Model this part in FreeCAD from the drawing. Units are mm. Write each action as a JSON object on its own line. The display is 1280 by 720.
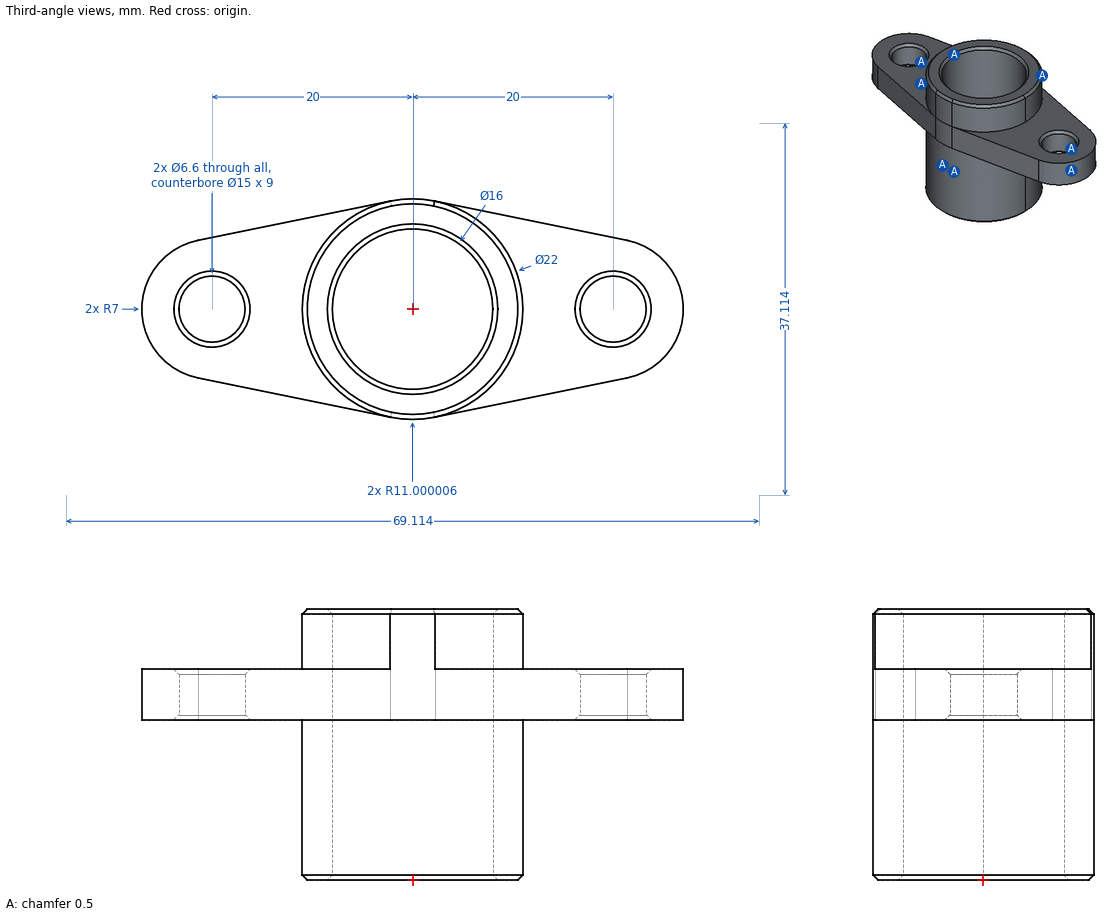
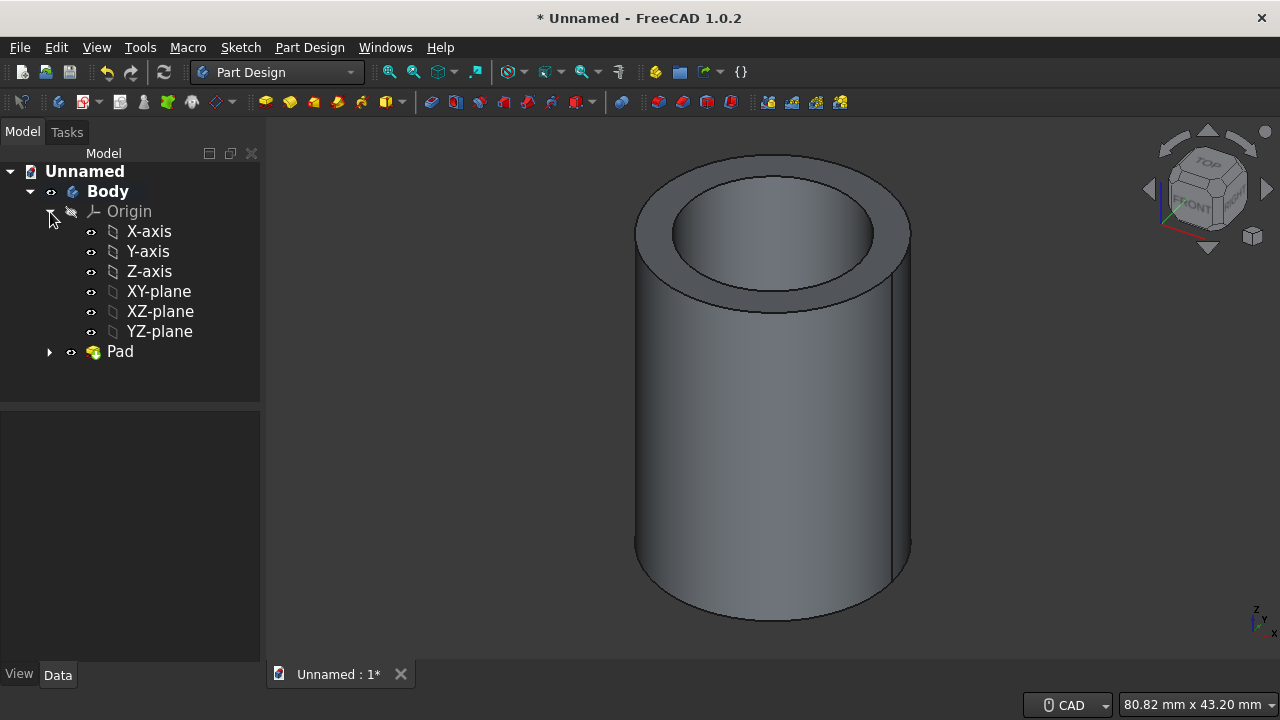
{"action": "left_click", "coordinate": [136, 292]}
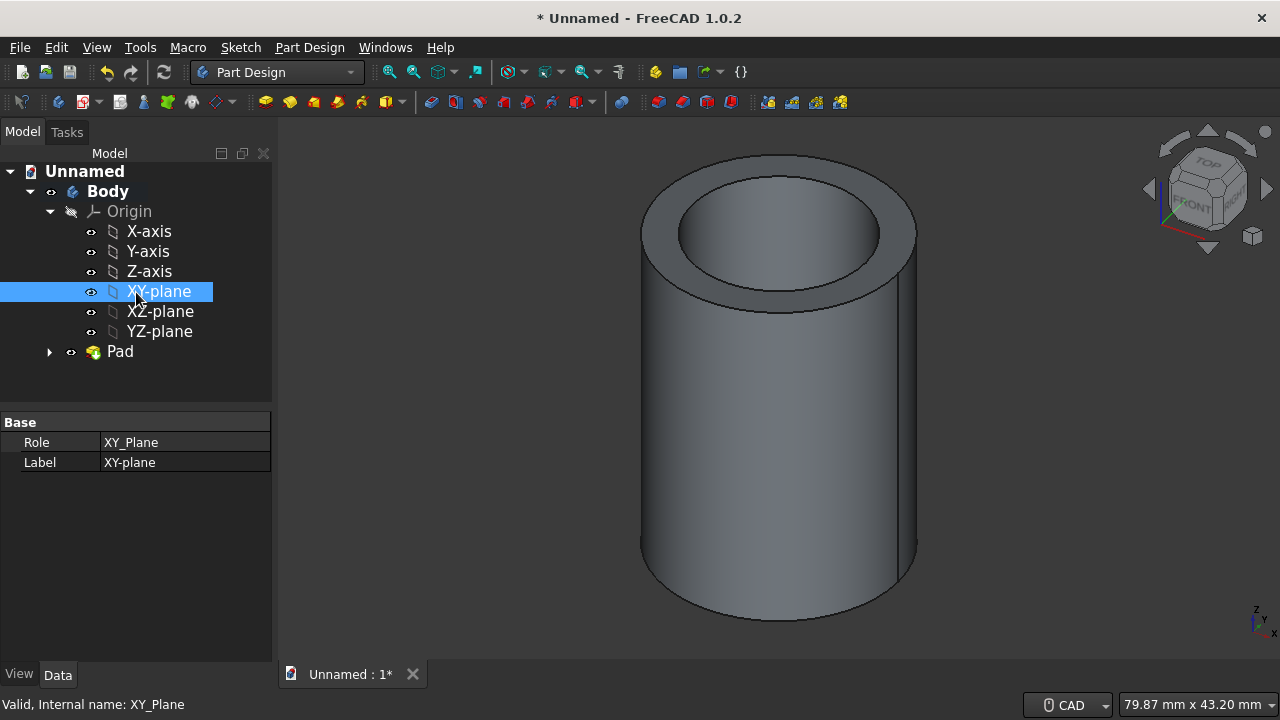
{"action": "left_click", "coordinate": [216, 102]}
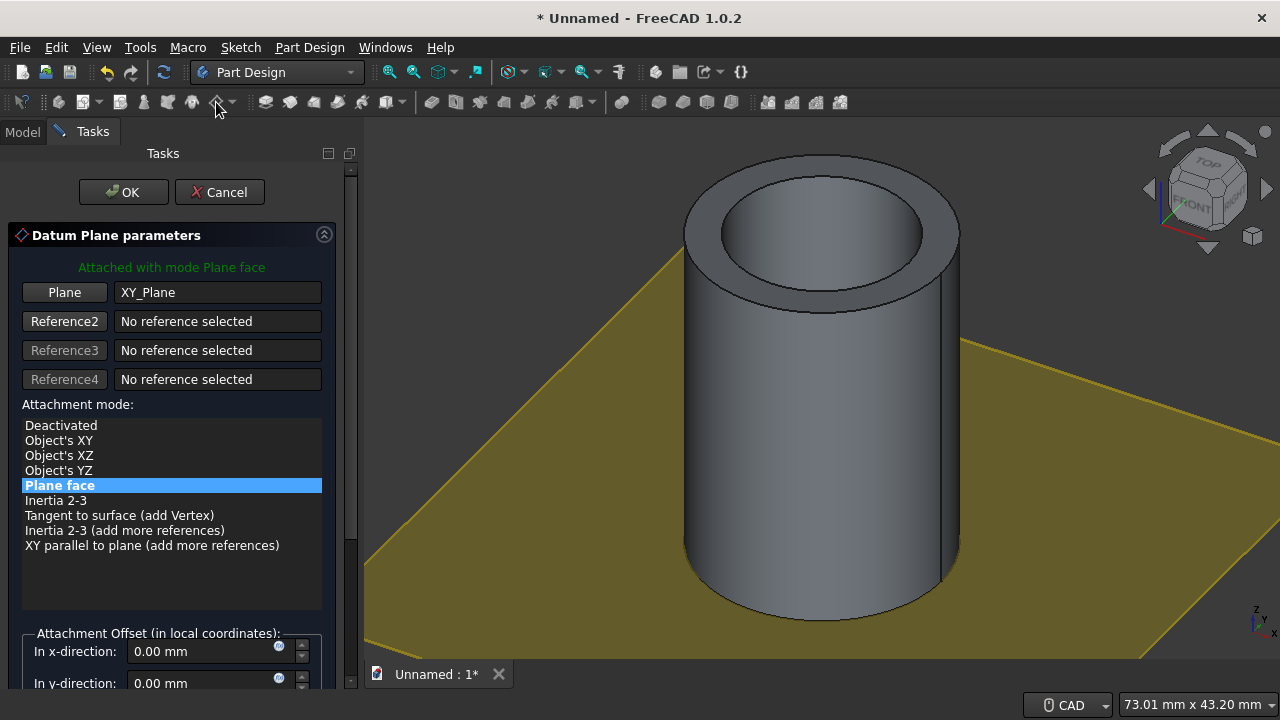
{"action": "scroll", "coordinate": [351, 426], "scroll_direction": "down", "scroll_amount": 2}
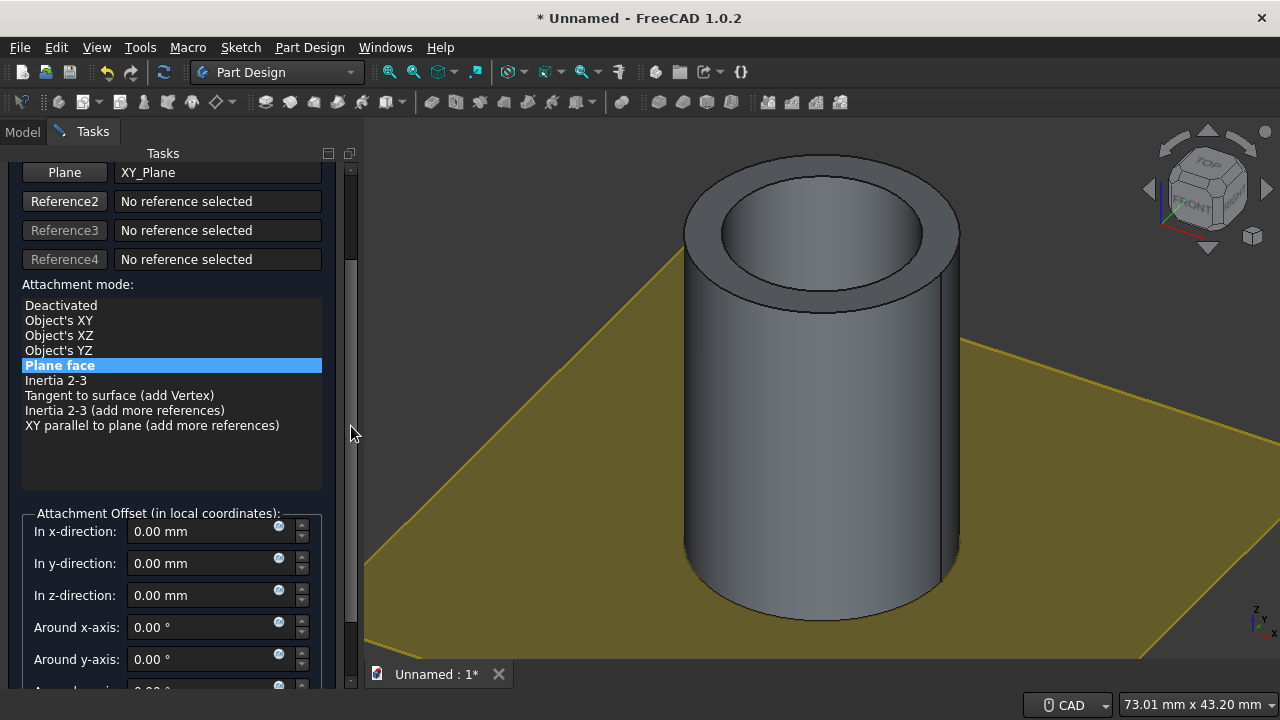
{"action": "triple_click", "coordinate": [210, 595]}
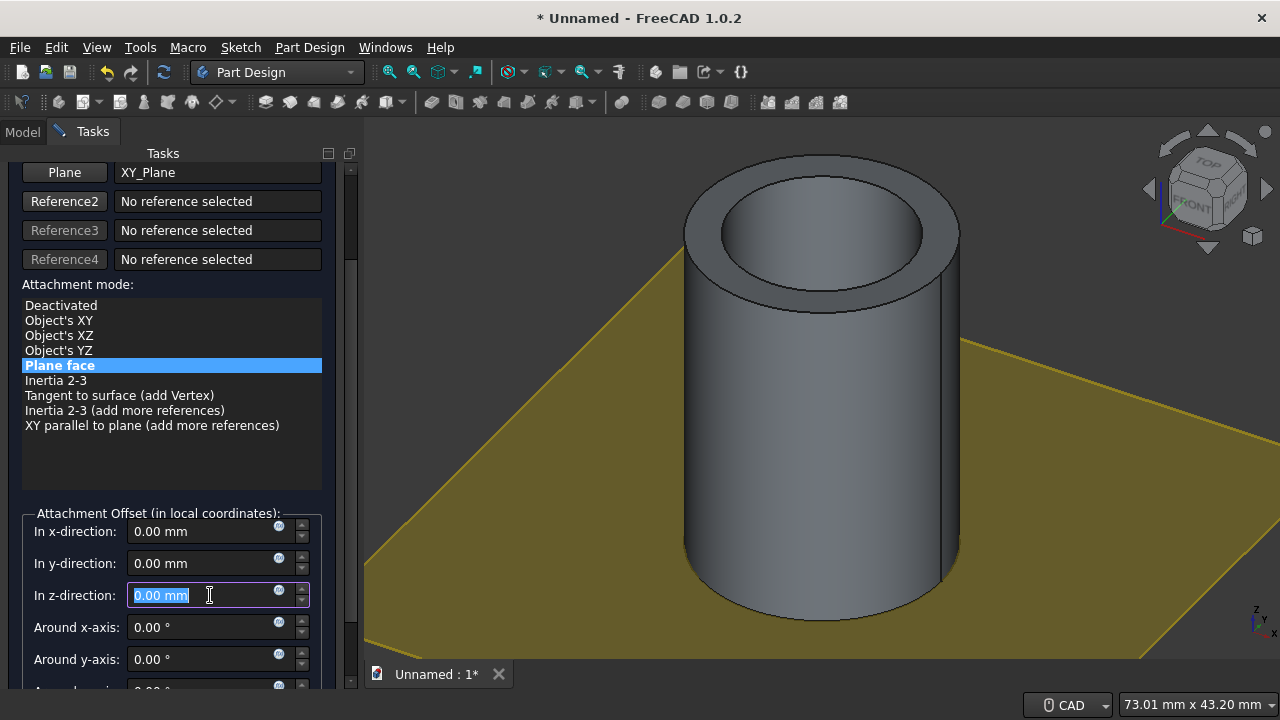
{"action": "type", "text": "16"}
{"action": "key", "text": "Tab"}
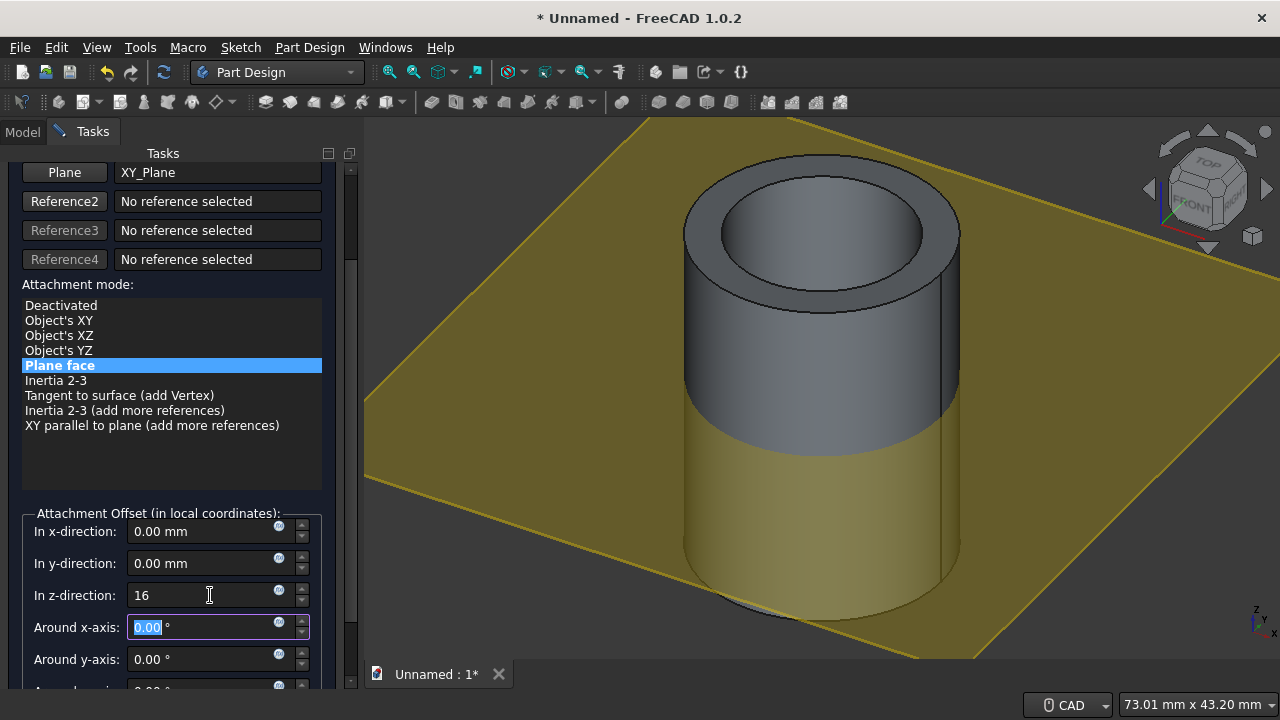
{"action": "scroll", "coordinate": [351, 426], "scroll_direction": "up", "scroll_amount": 3}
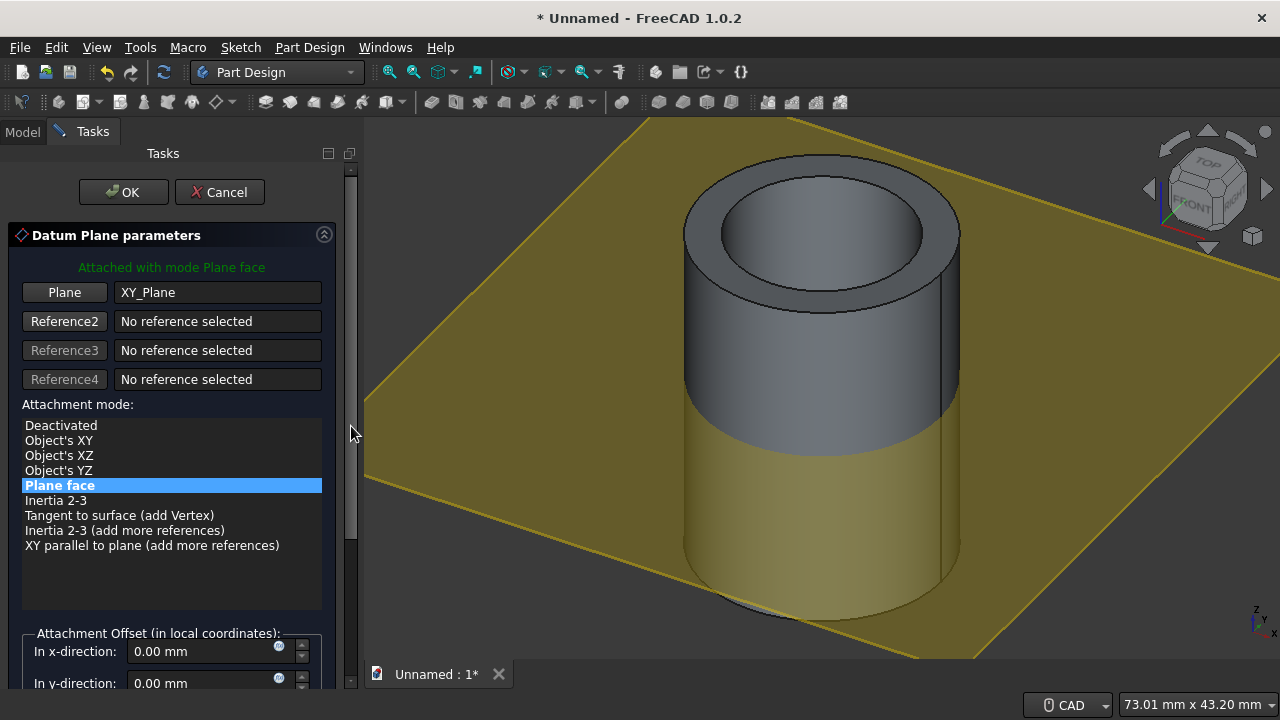
{"action": "left_click", "coordinate": [124, 192]}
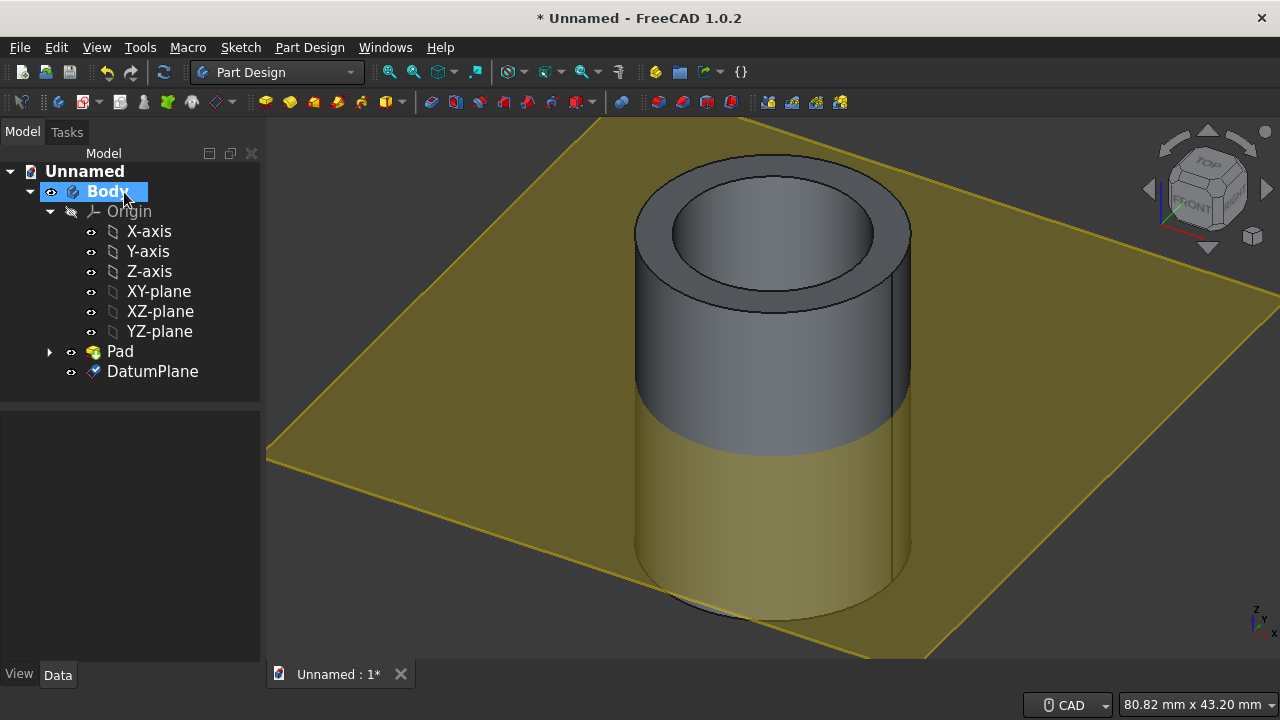
{"action": "left_click", "coordinate": [116, 372]}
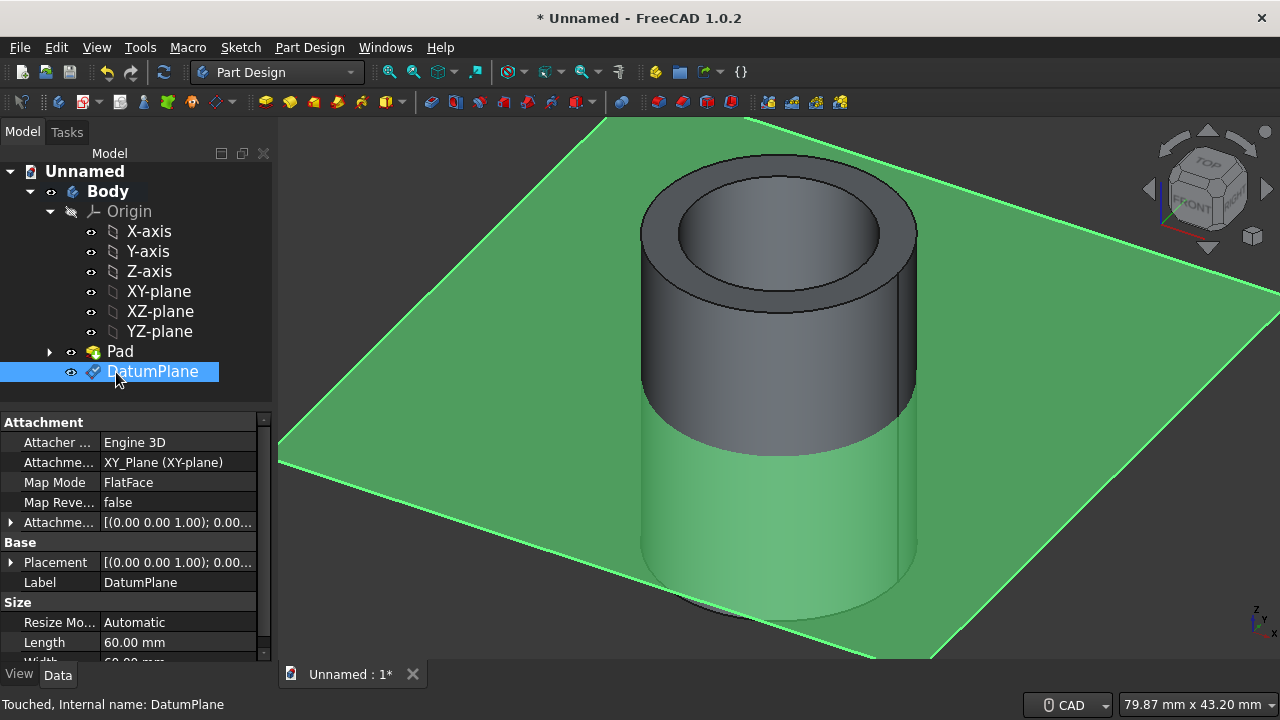
{"action": "left_click", "coordinate": [84, 102]}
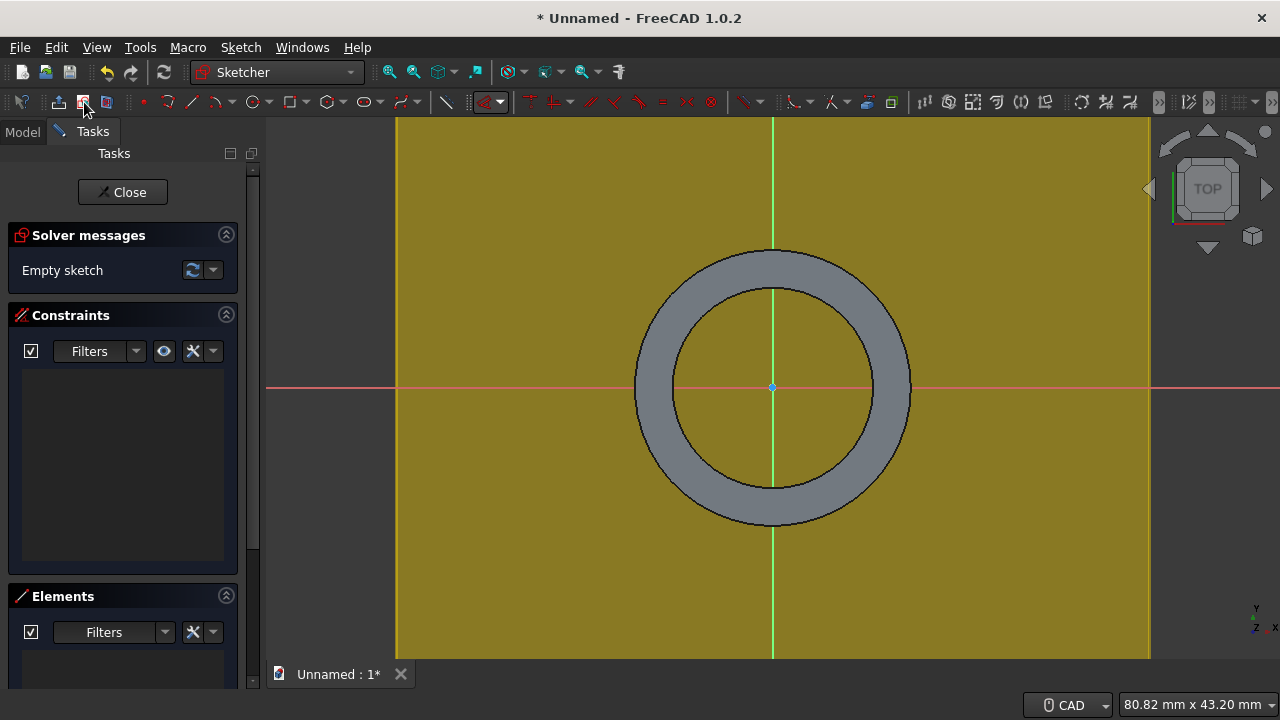
{"action": "left_click", "coordinate": [108, 102]}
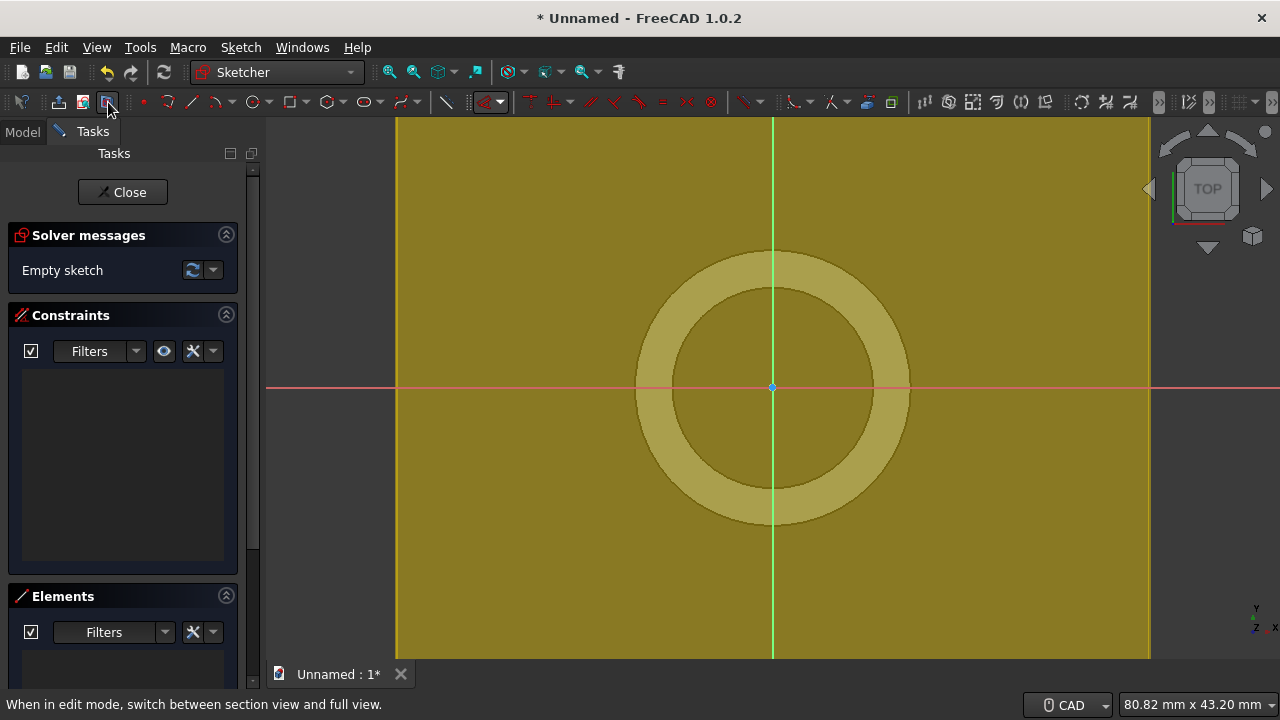
{"action": "scroll", "coordinate": [396, 388], "scroll_direction": "down", "scroll_amount": 1}